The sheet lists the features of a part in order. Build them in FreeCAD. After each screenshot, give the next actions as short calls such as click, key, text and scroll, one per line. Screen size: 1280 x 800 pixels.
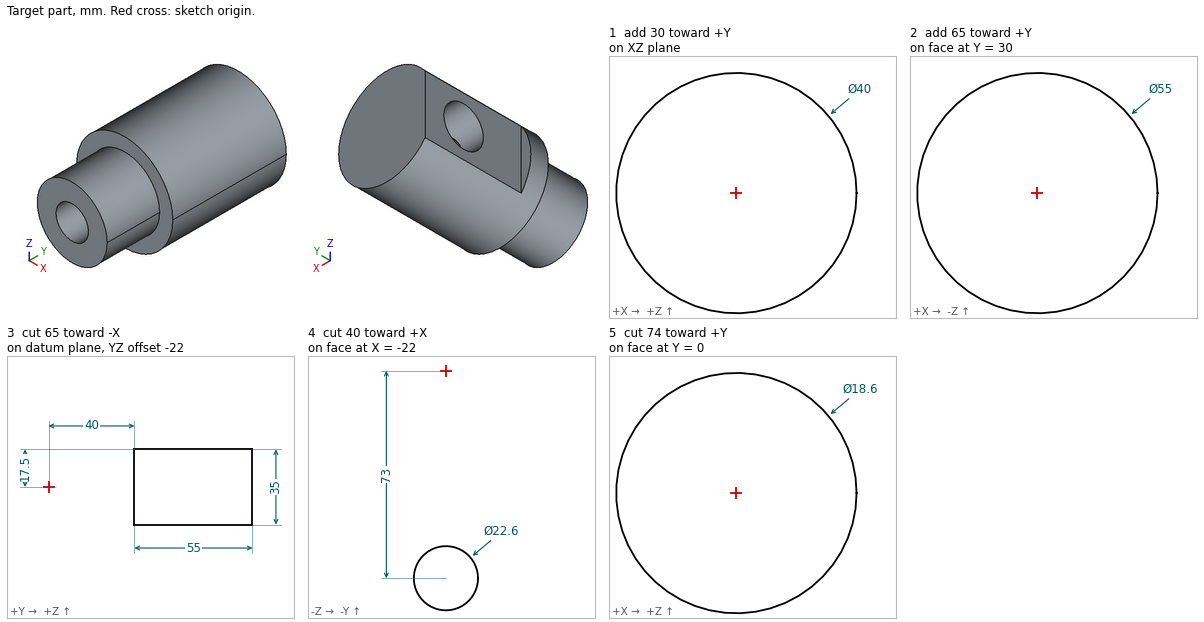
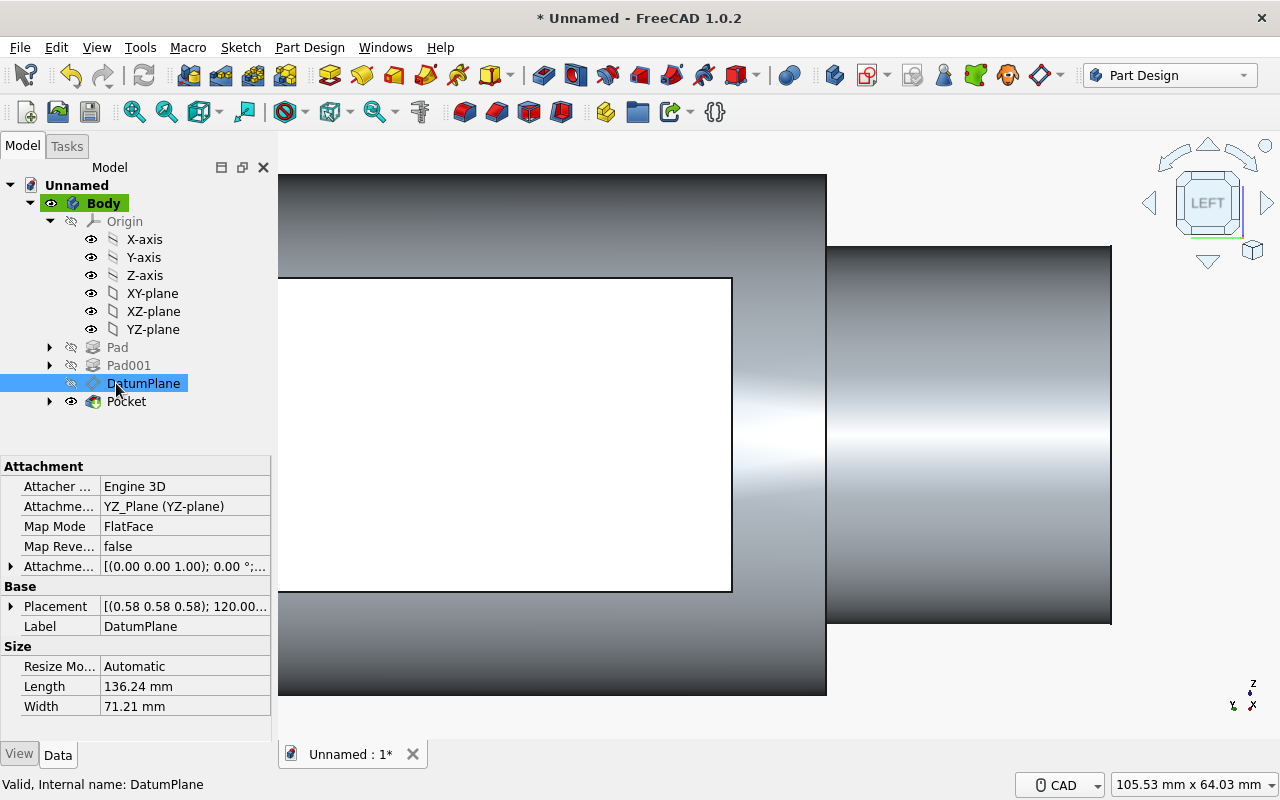
click(136, 112)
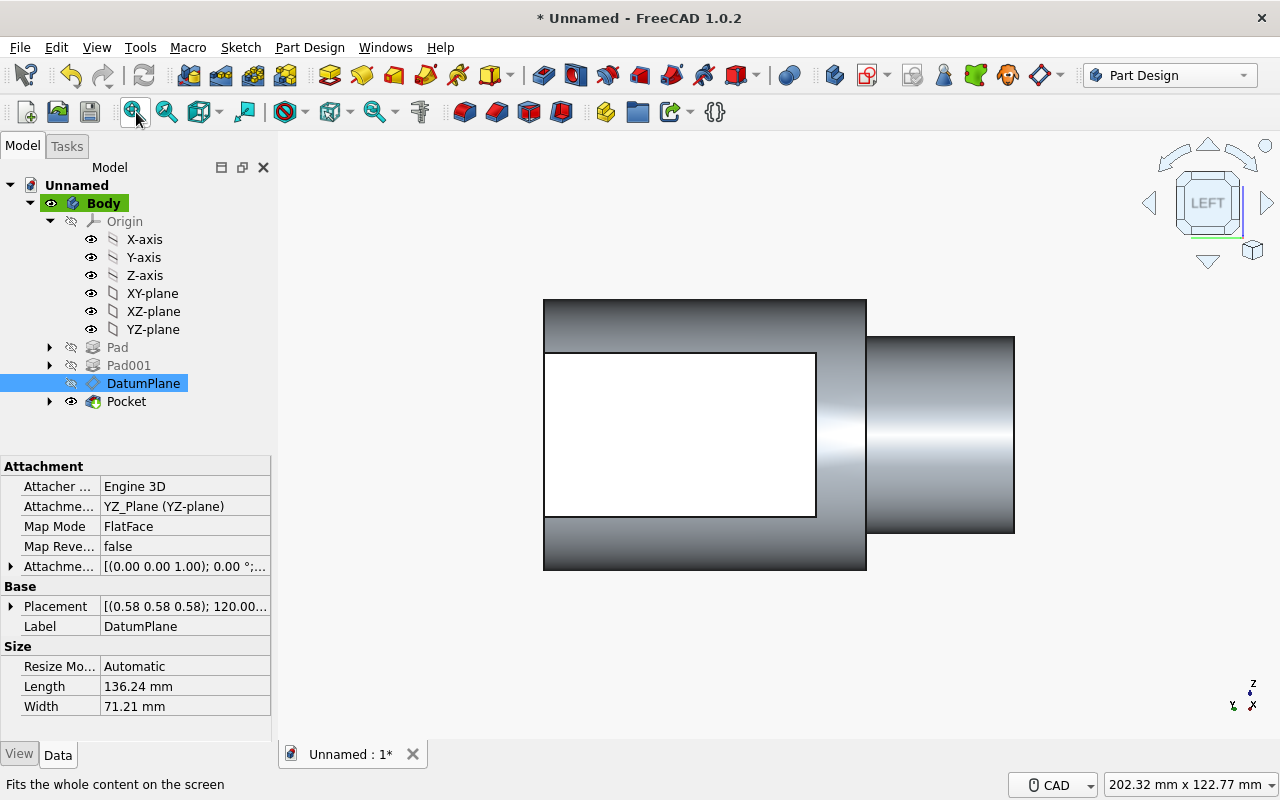
click(680, 434)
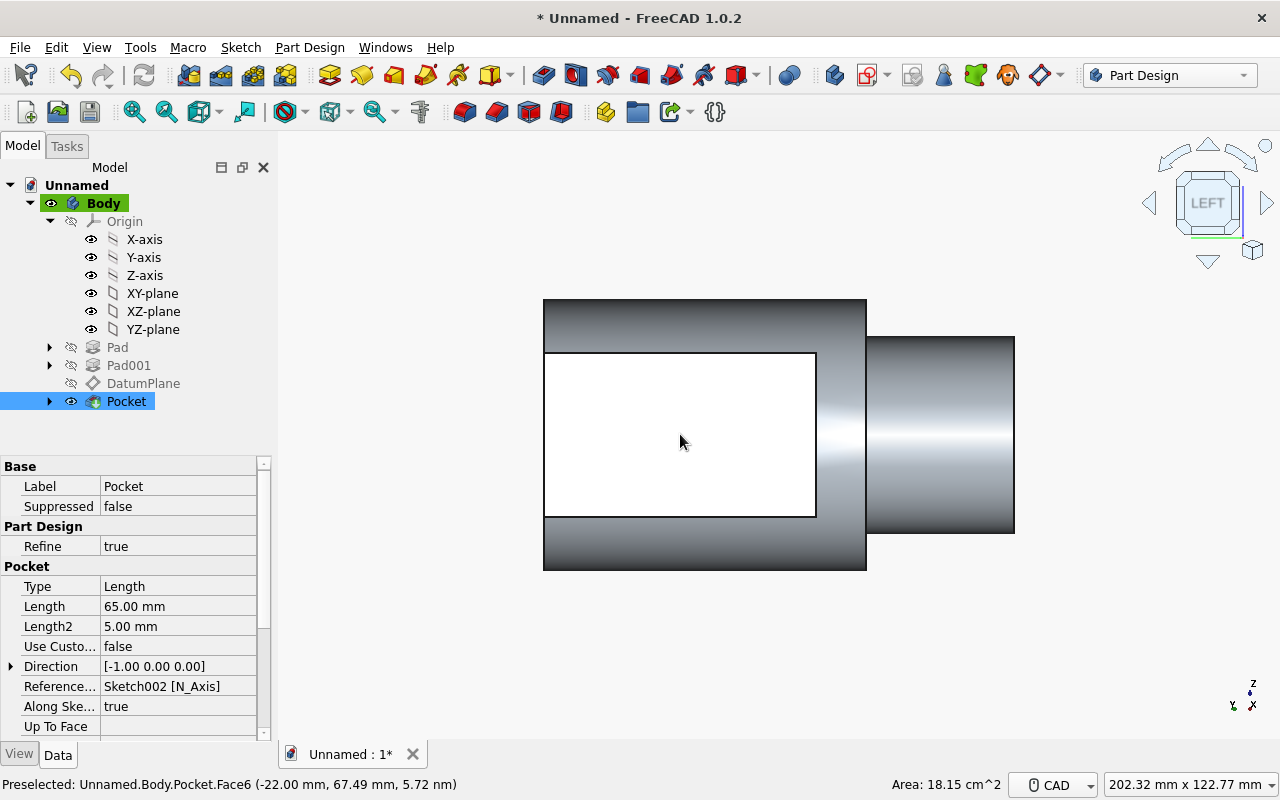
click(868, 76)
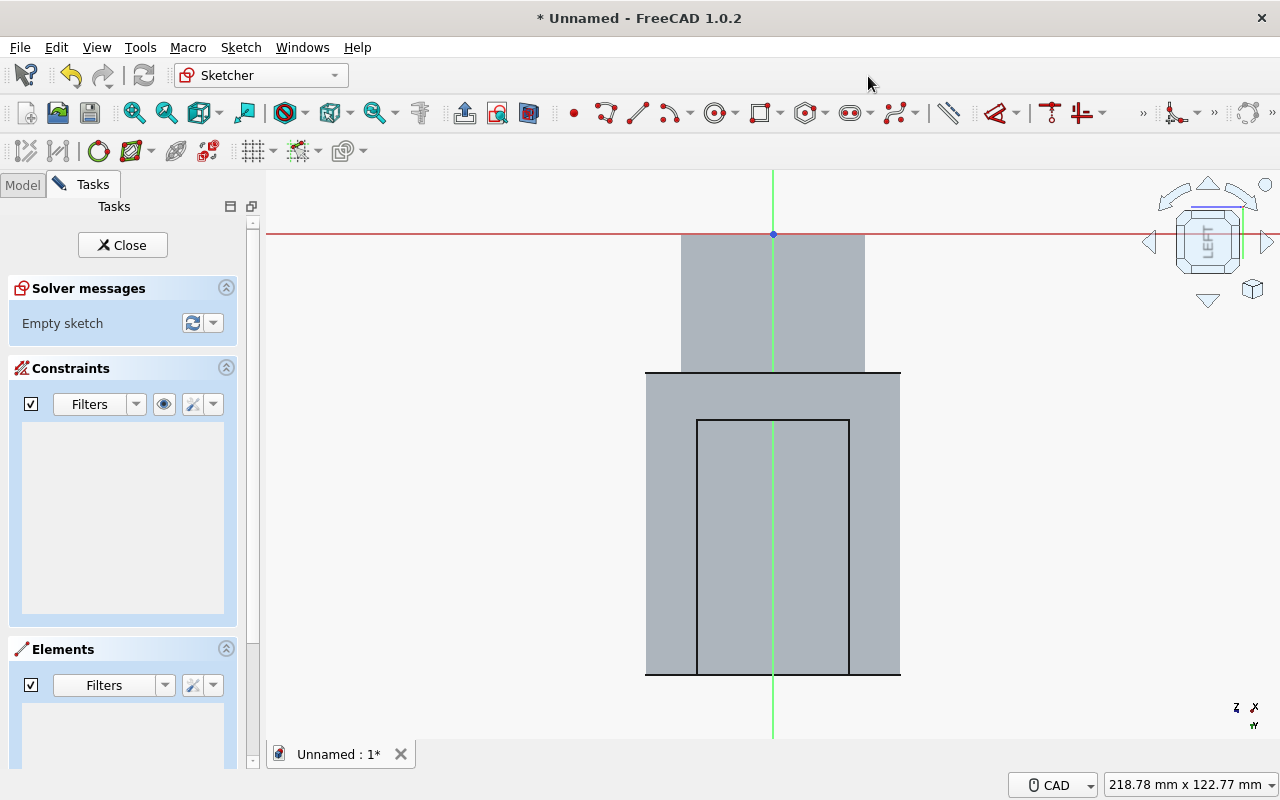
scroll(803, 624, up, 6)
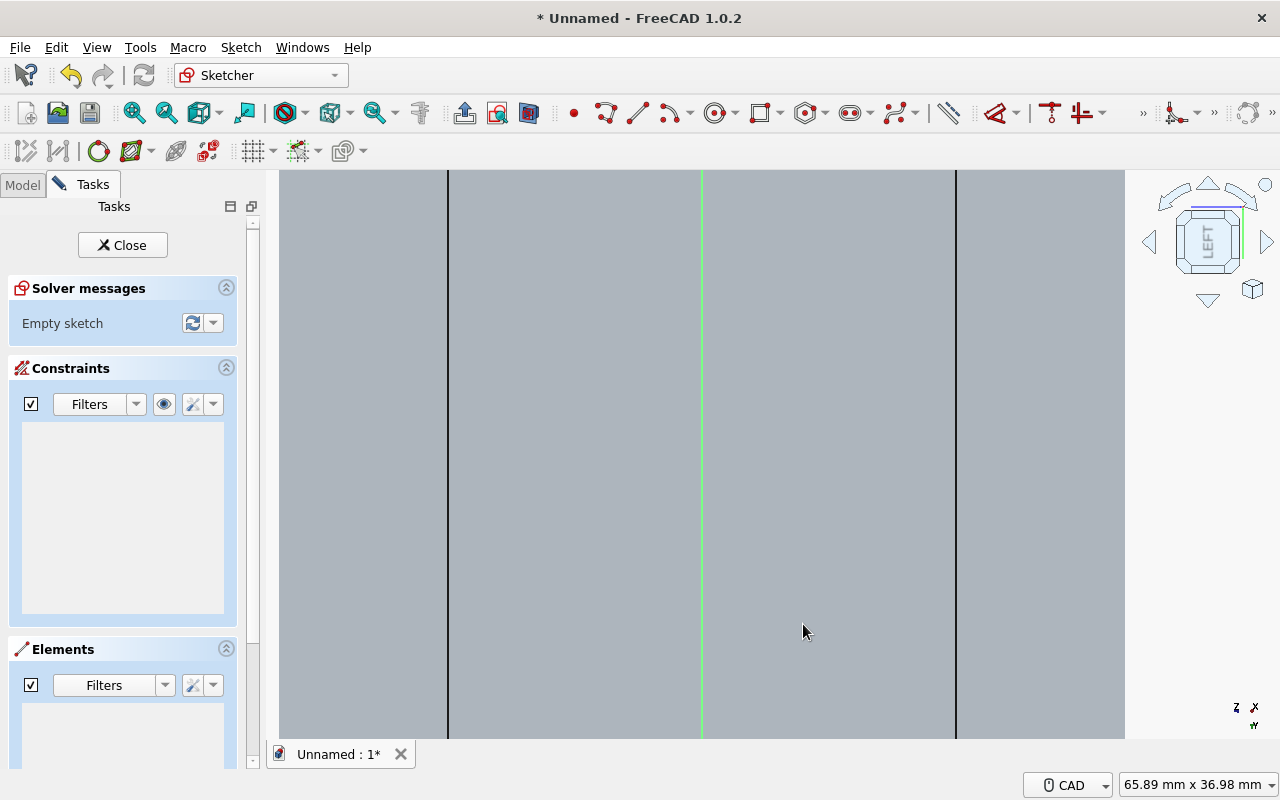
key(g)
key(c)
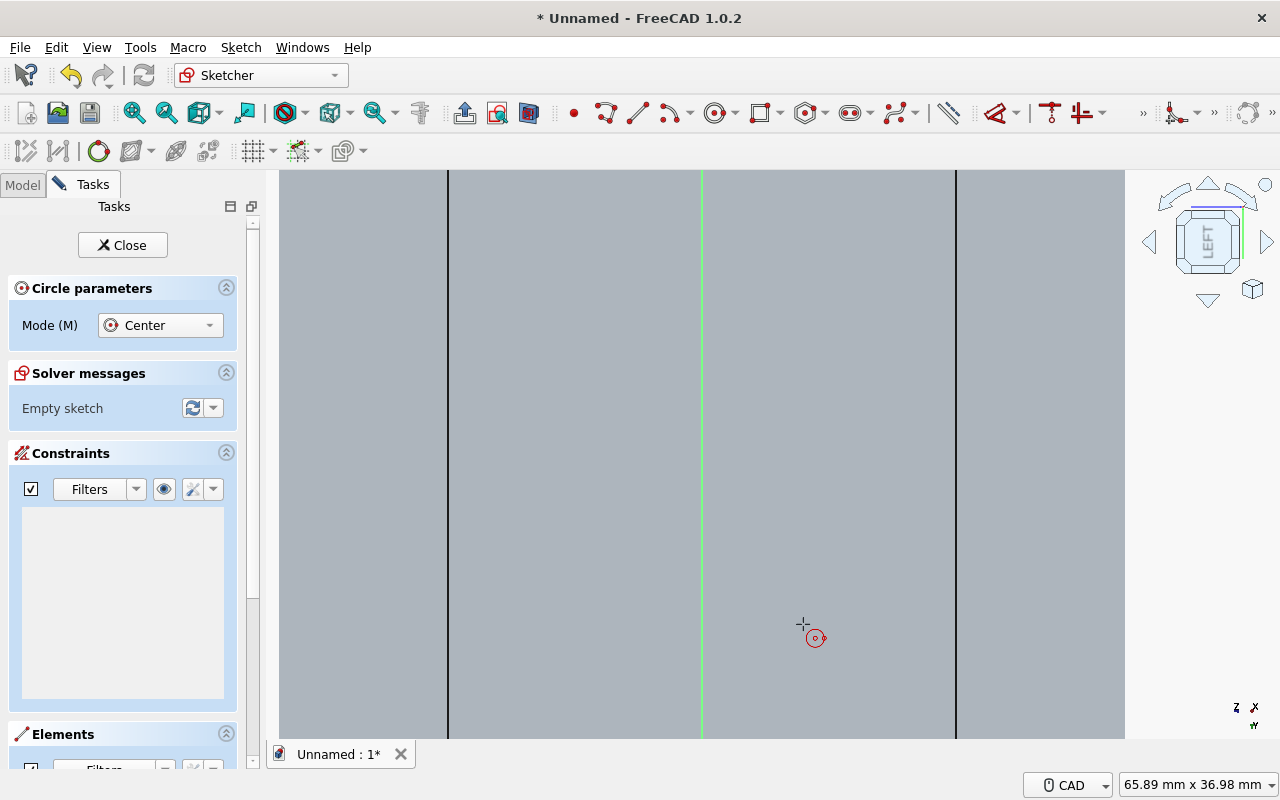
click(702, 452)
move(825, 329)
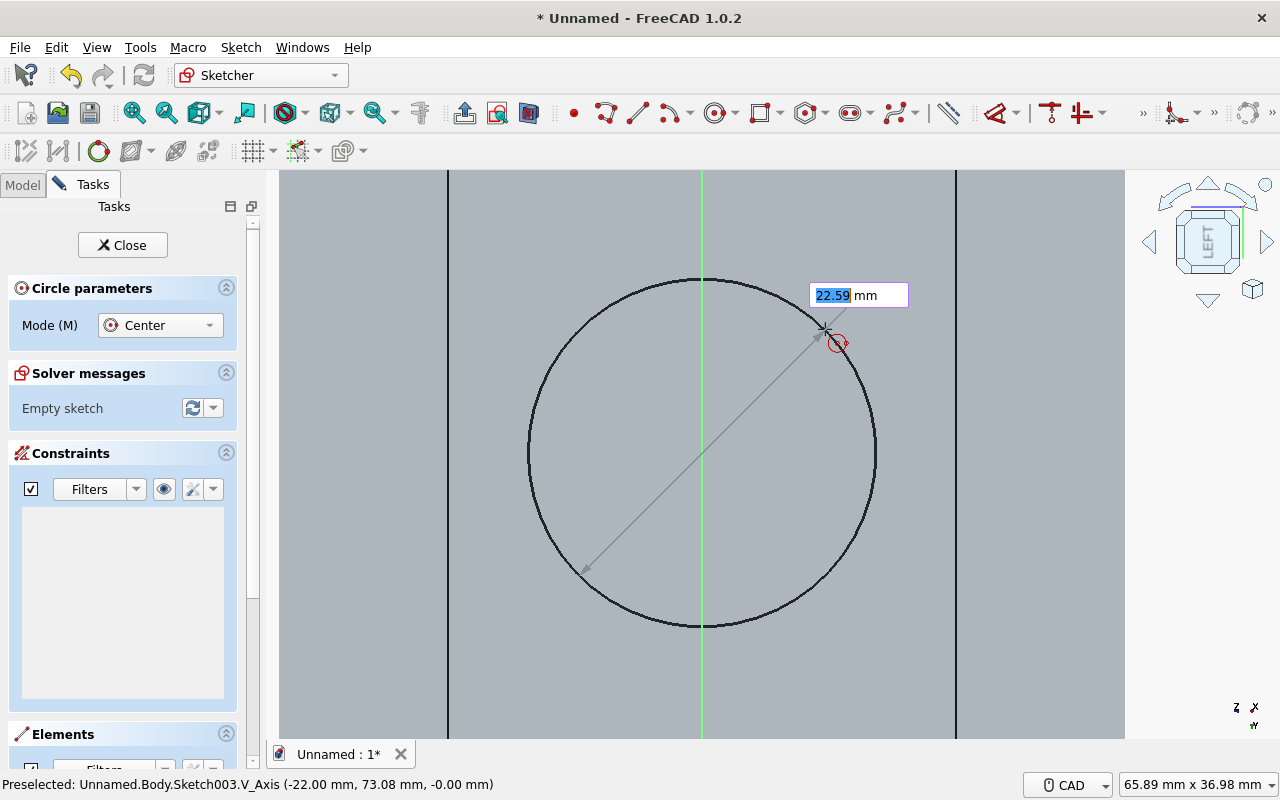
text(22.6)
key(Return)
key(Escape)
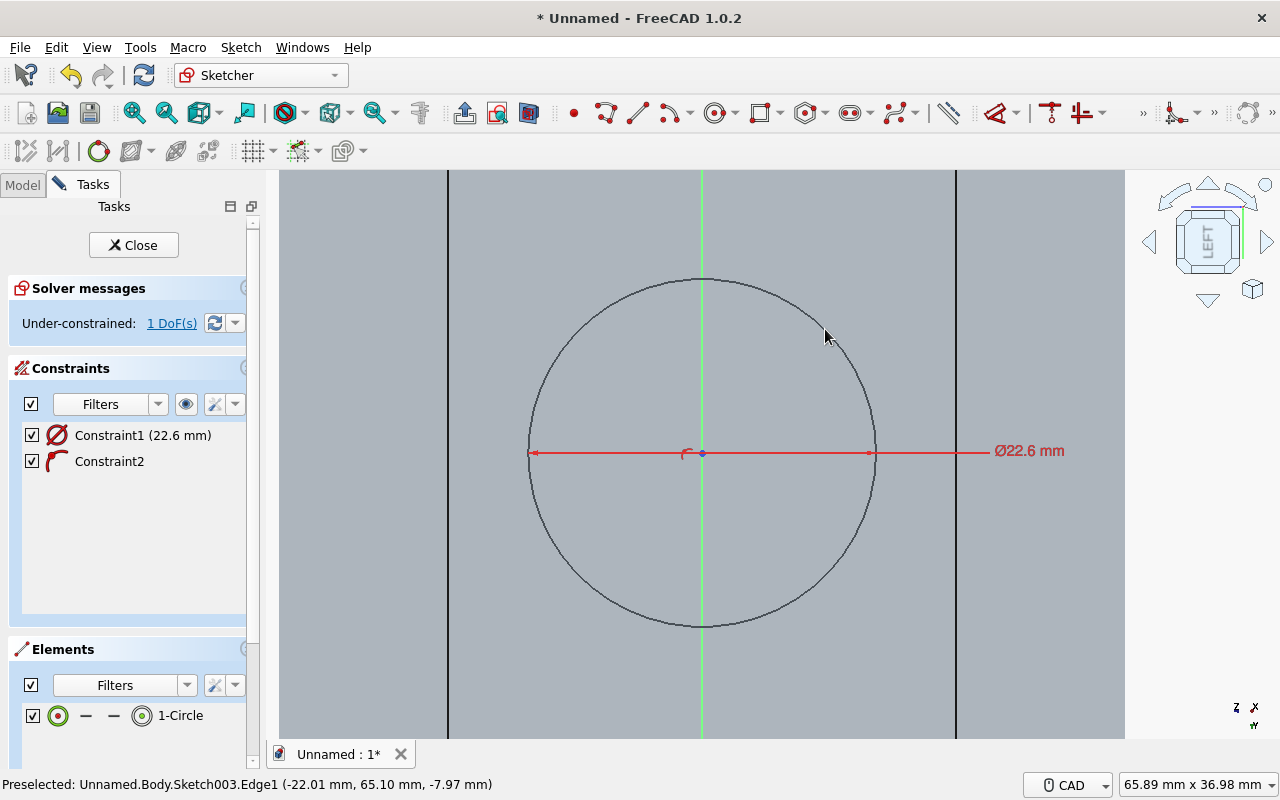
click(996, 114)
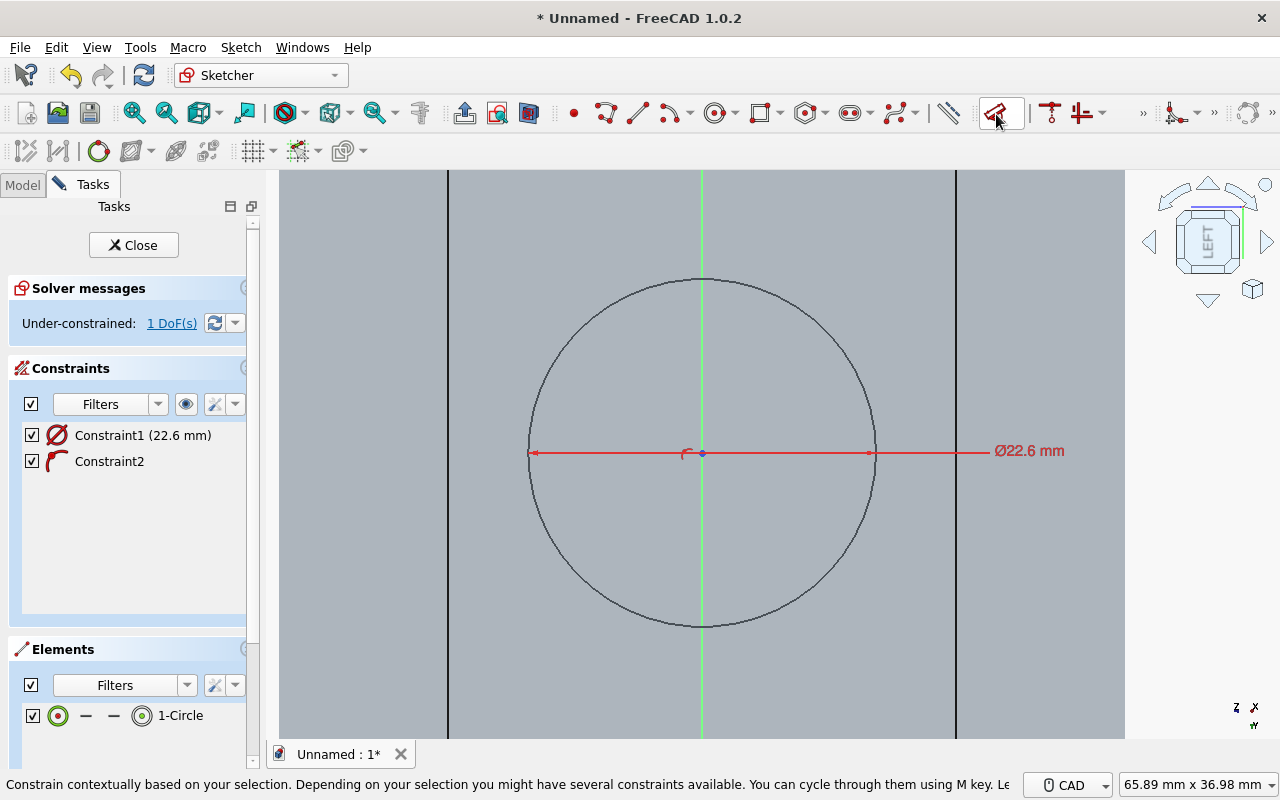
click(702, 453)
click(736, 326)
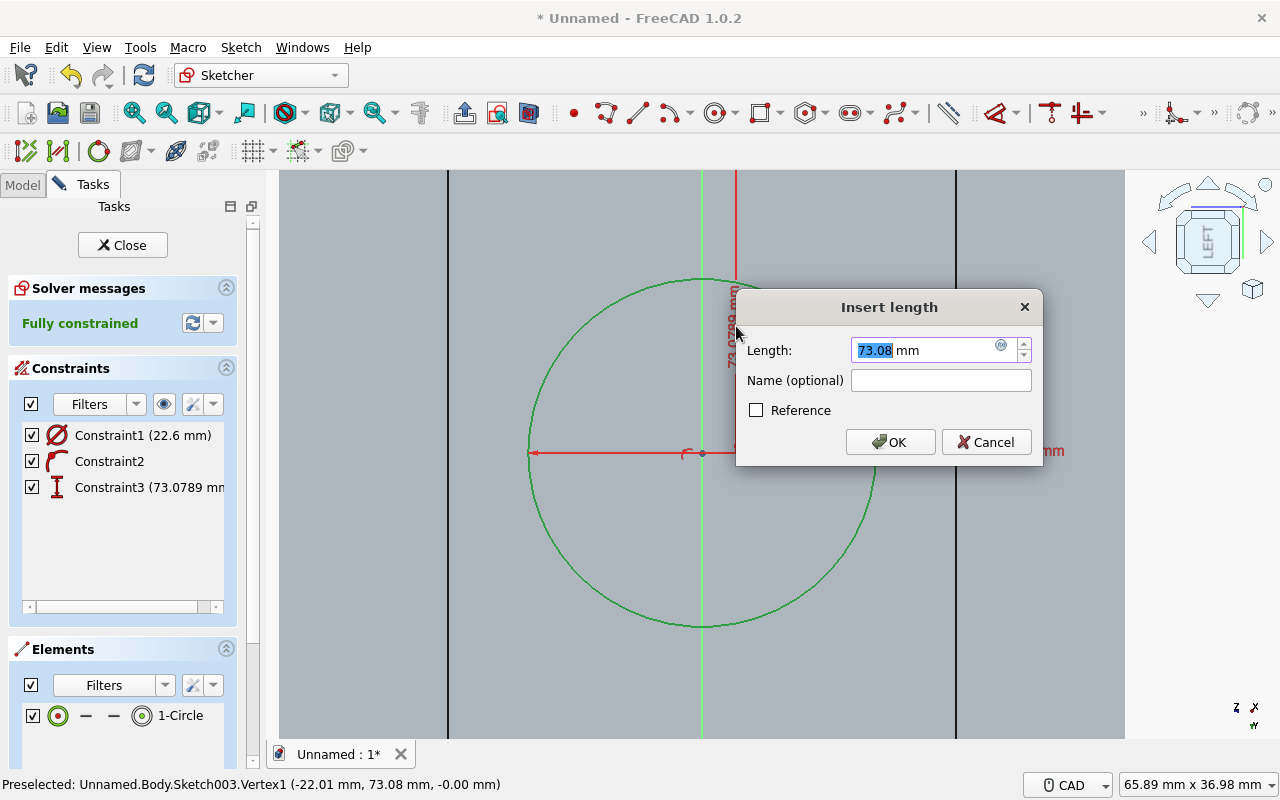
text(73)
key(Return)
key(Escape)